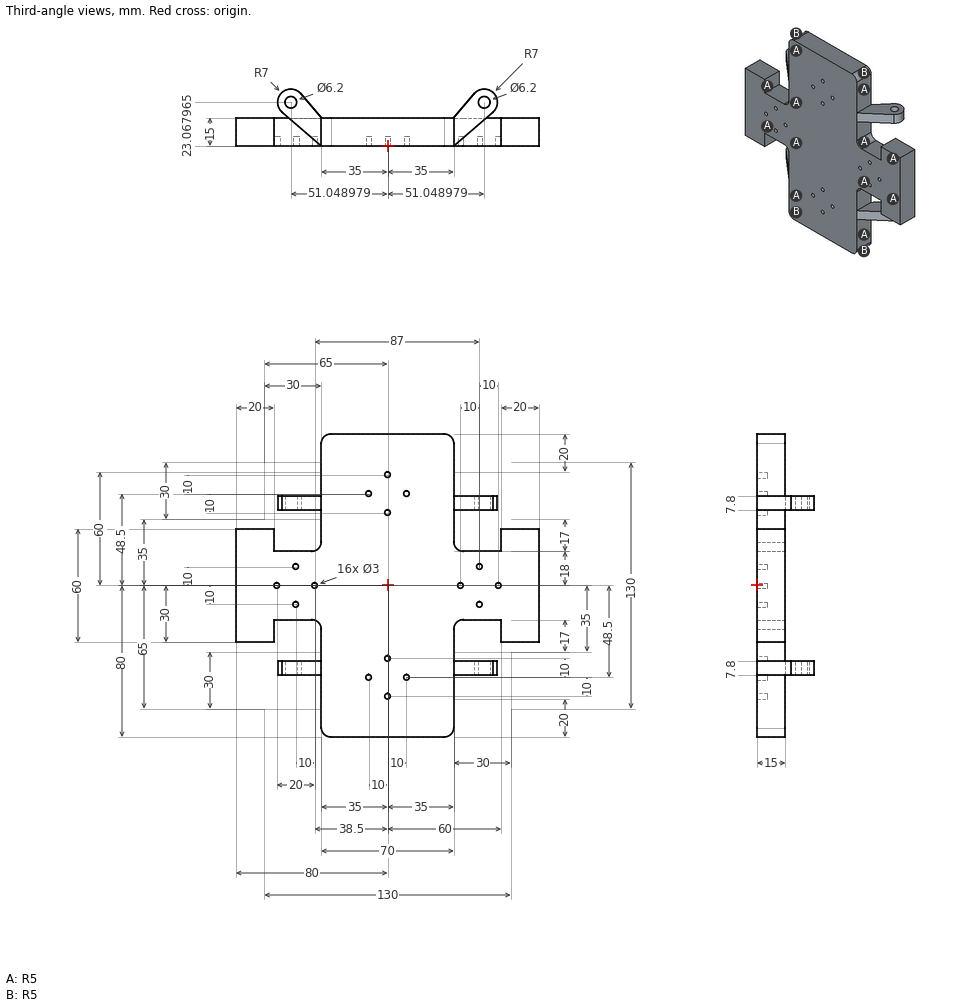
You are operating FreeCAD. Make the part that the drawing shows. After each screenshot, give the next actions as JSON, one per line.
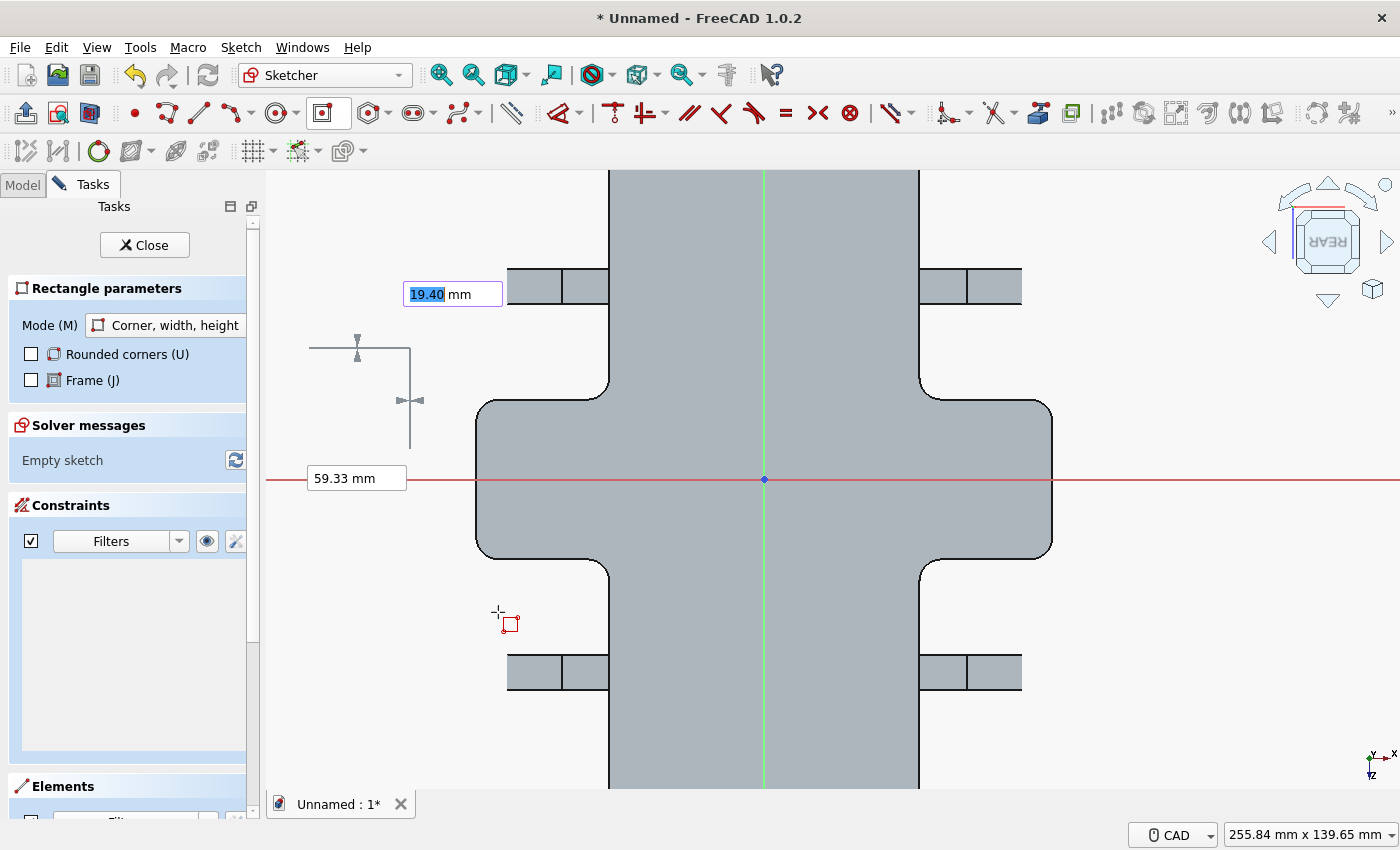
{"action": "type", "text": "20"}
{"action": "key", "text": "Tab"}
{"action": "type", "text": "60"}
{"action": "key", "text": "Return"}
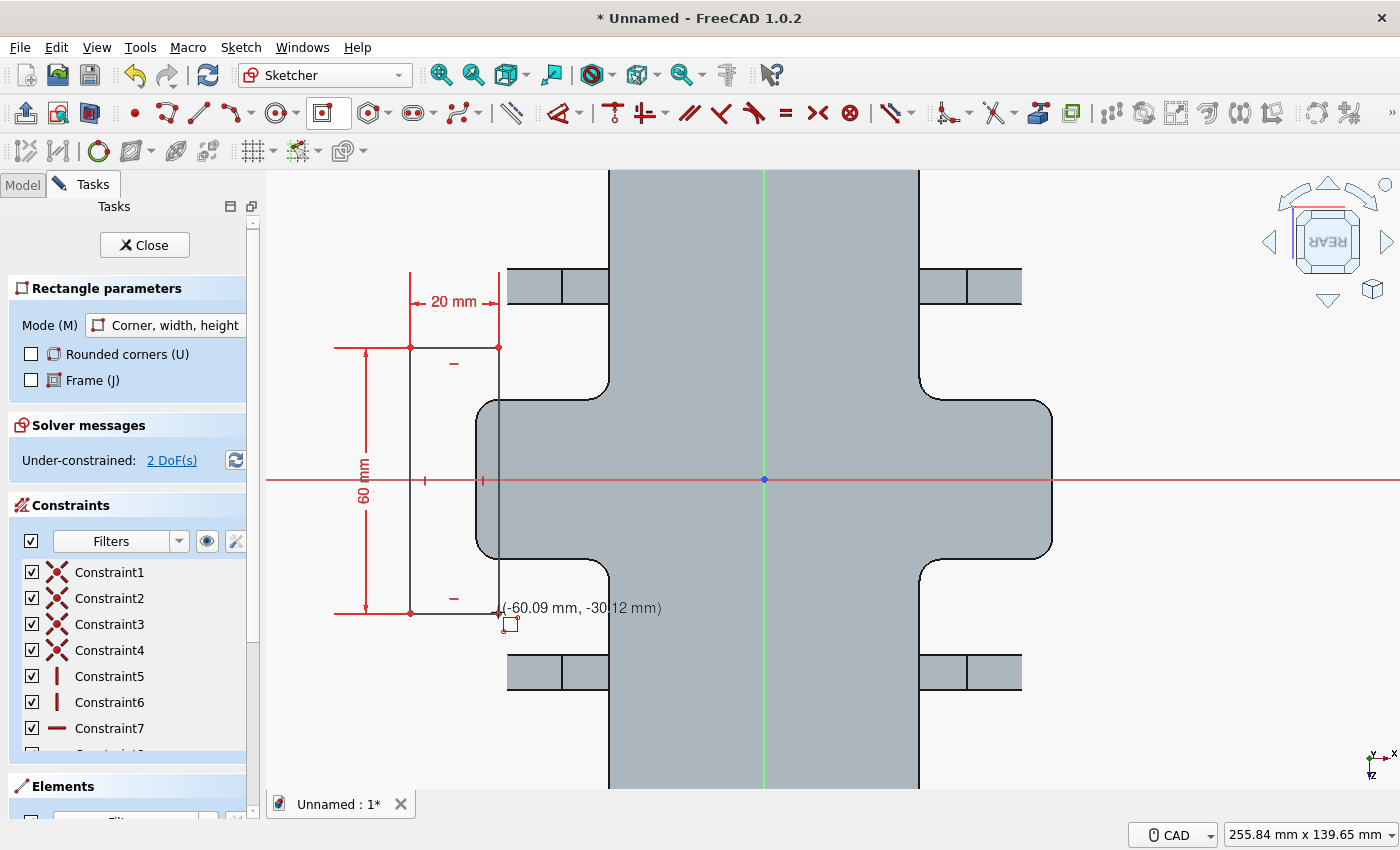
{"action": "left_click", "coordinate": [1030, 347]}
{"action": "mouse_move", "coordinate": [1119, 612]}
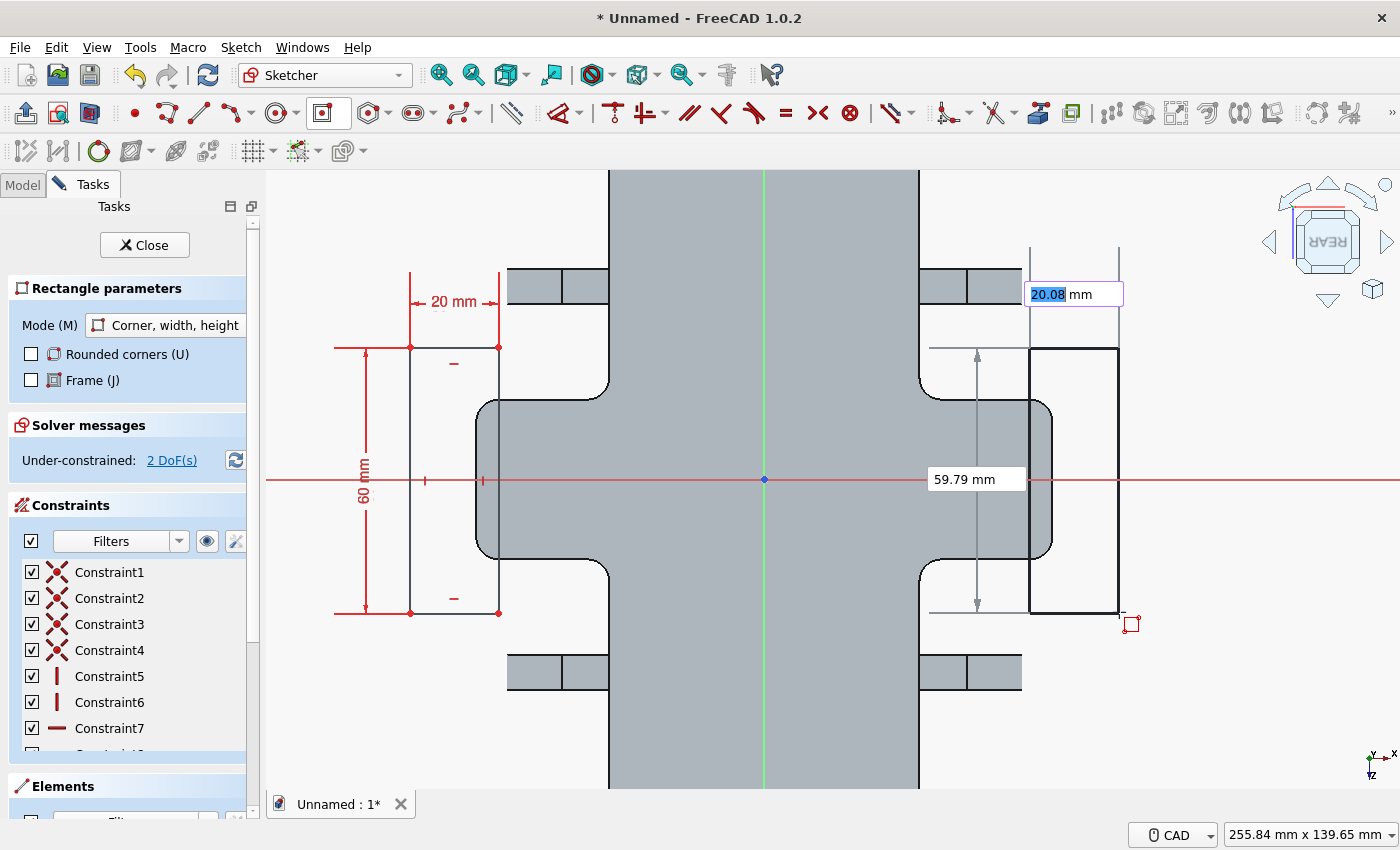
{"action": "type", "text": "20"}
{"action": "key", "text": "Tab"}
{"action": "type", "text": "60"}
{"action": "key", "text": "Return"}
{"action": "key", "text": "Escape"}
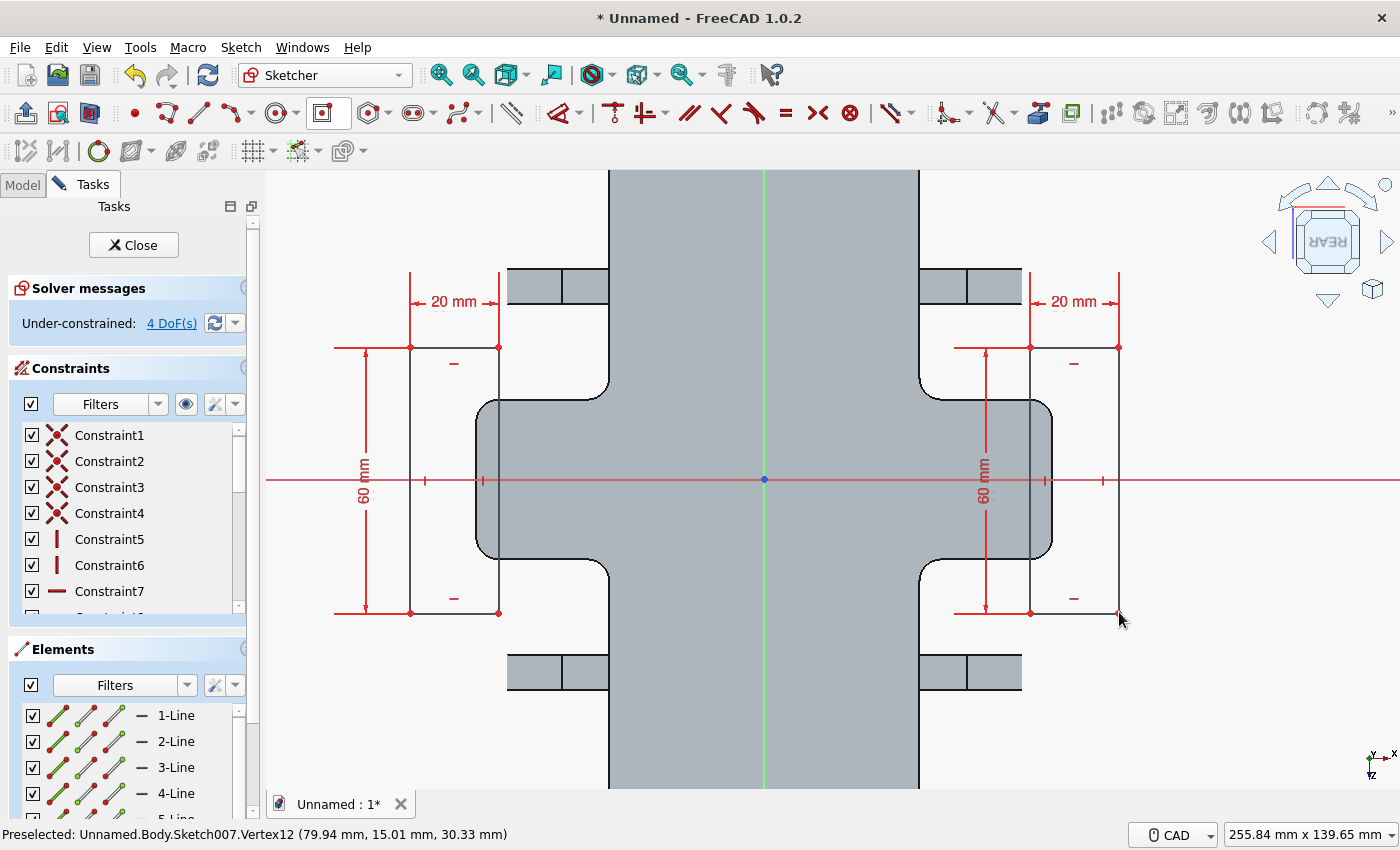
{"action": "key", "text": "d"}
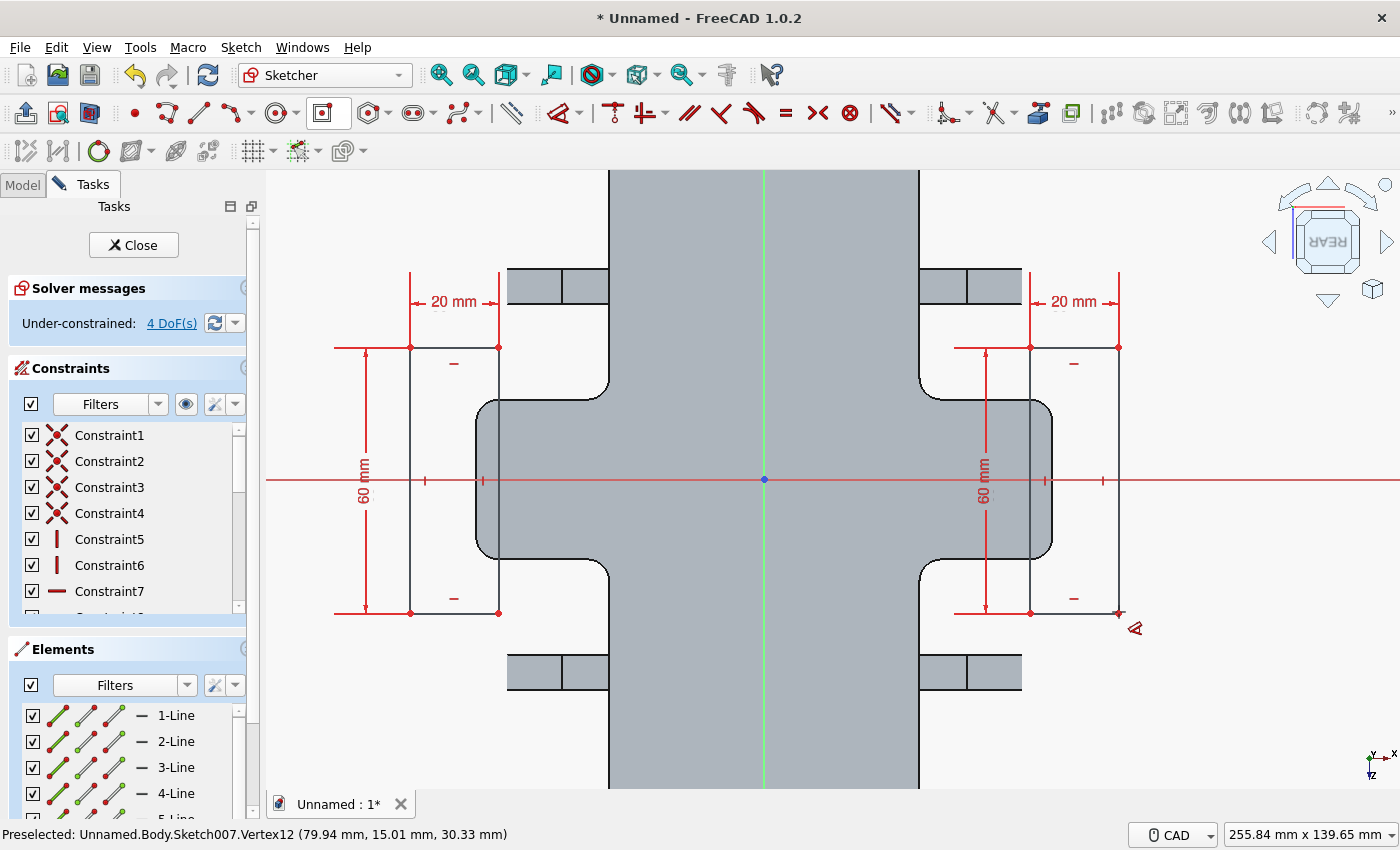
{"action": "left_click", "coordinate": [410, 348]}
{"action": "left_click", "coordinate": [587, 314]}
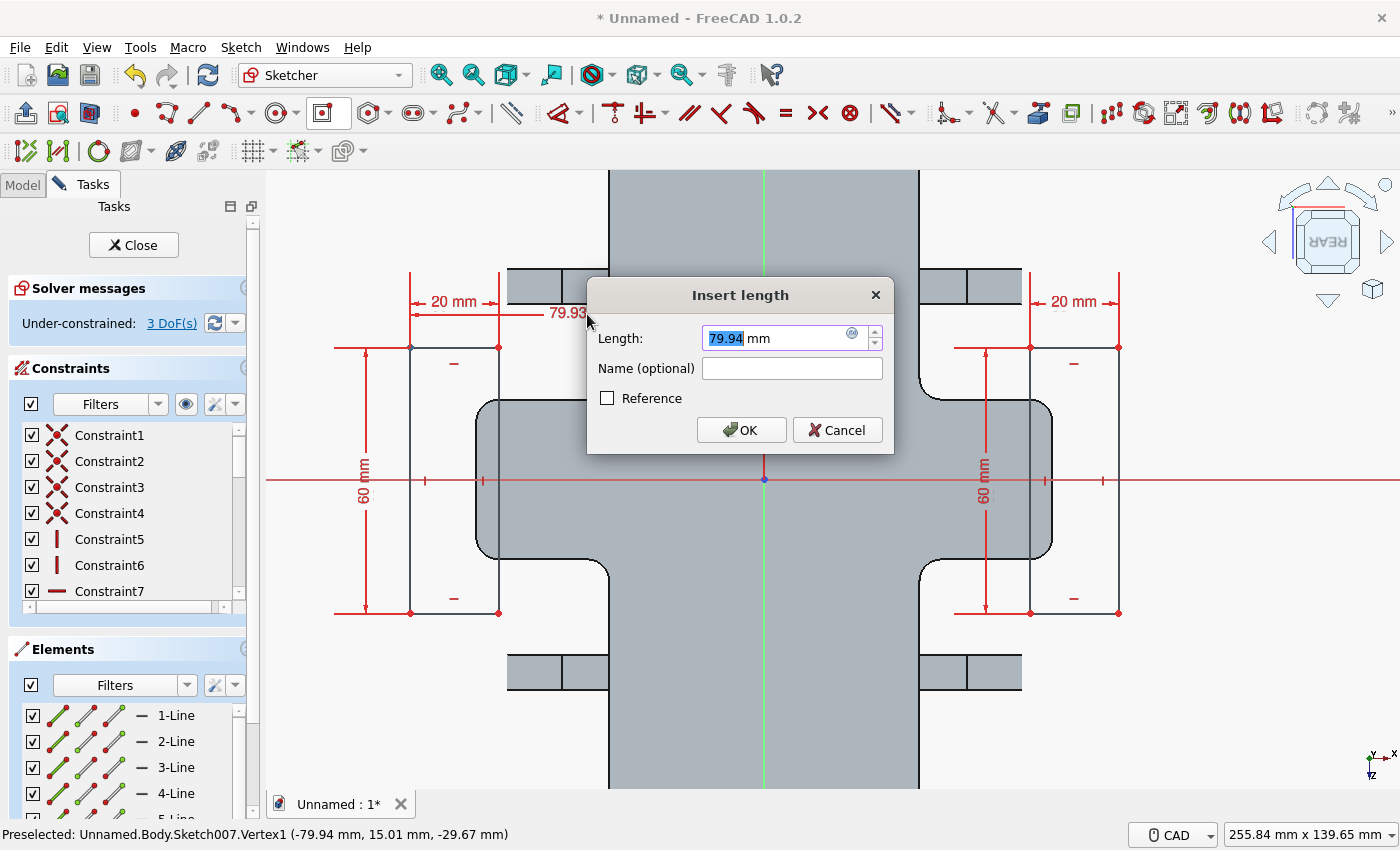
{"action": "type", "text": "80"}
{"action": "key", "text": "Return"}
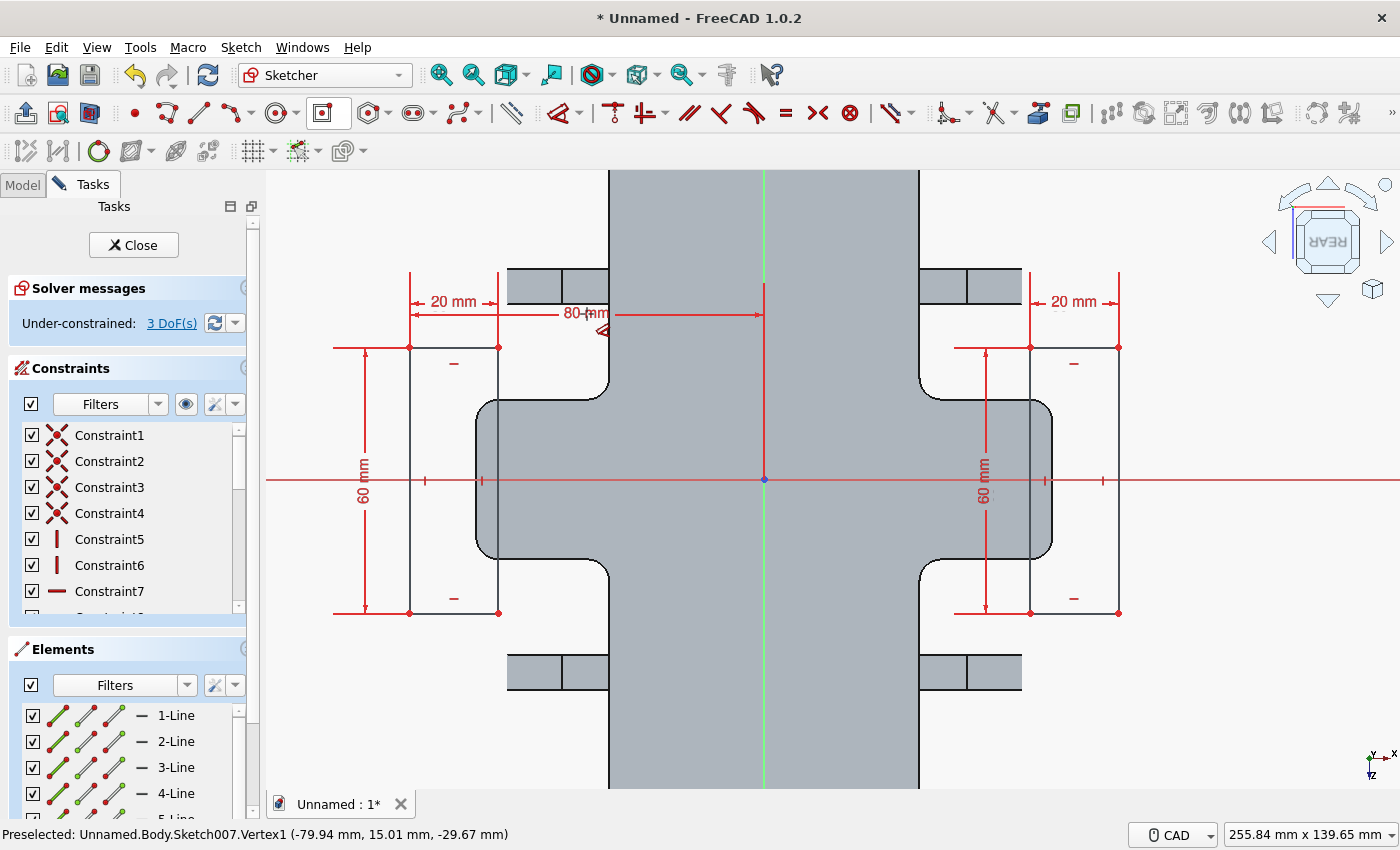
{"action": "left_click", "coordinate": [410, 348]}
{"action": "left_click", "coordinate": [376, 414]}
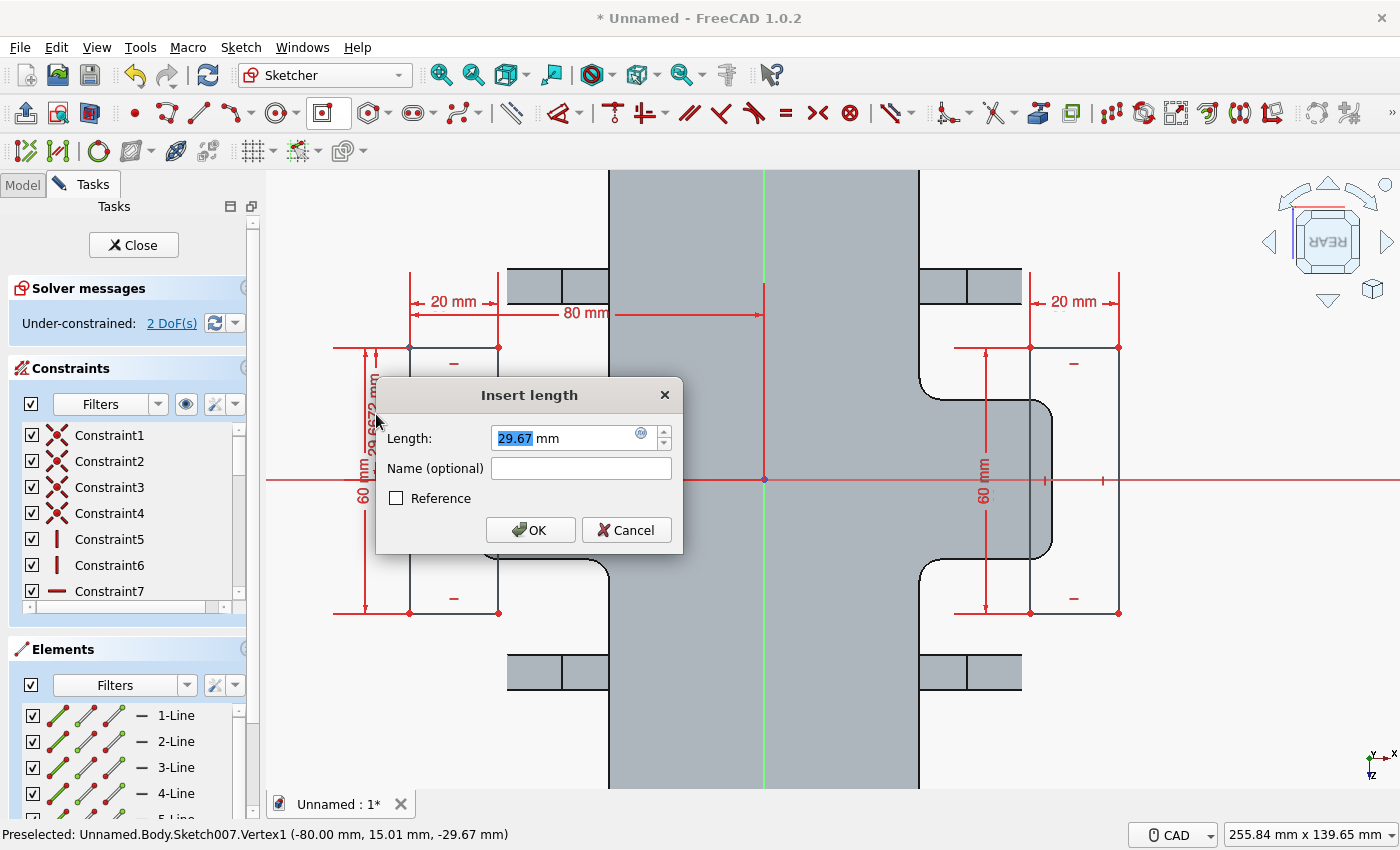
{"action": "type", "text": "30"}
{"action": "key", "text": "Return"}